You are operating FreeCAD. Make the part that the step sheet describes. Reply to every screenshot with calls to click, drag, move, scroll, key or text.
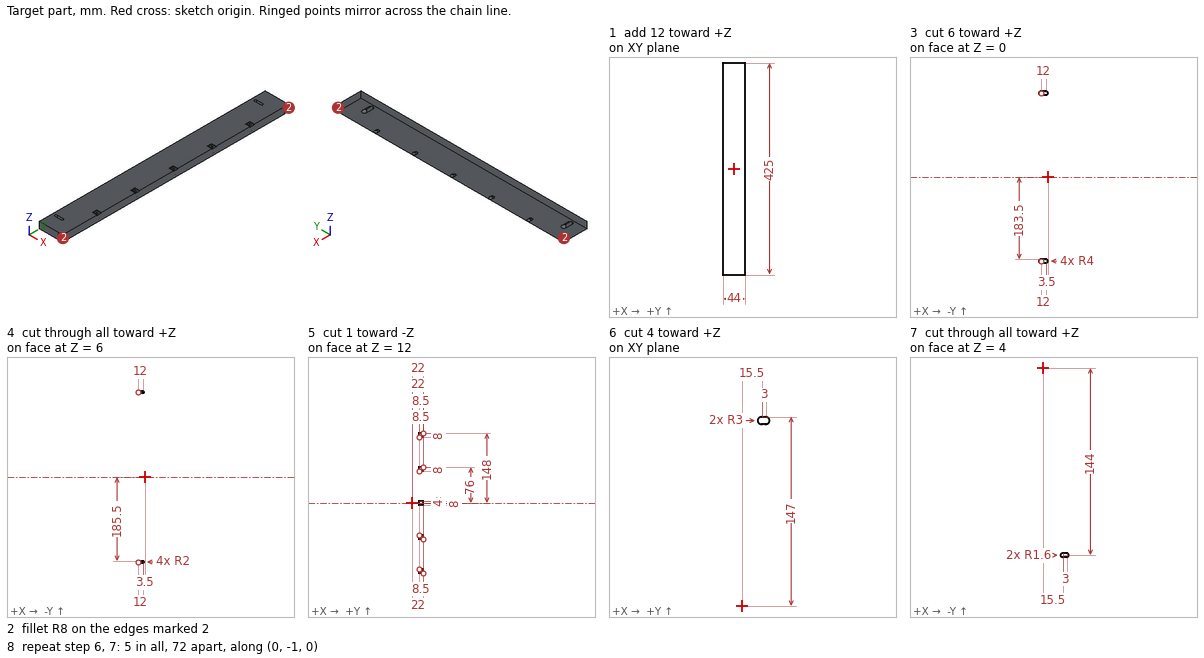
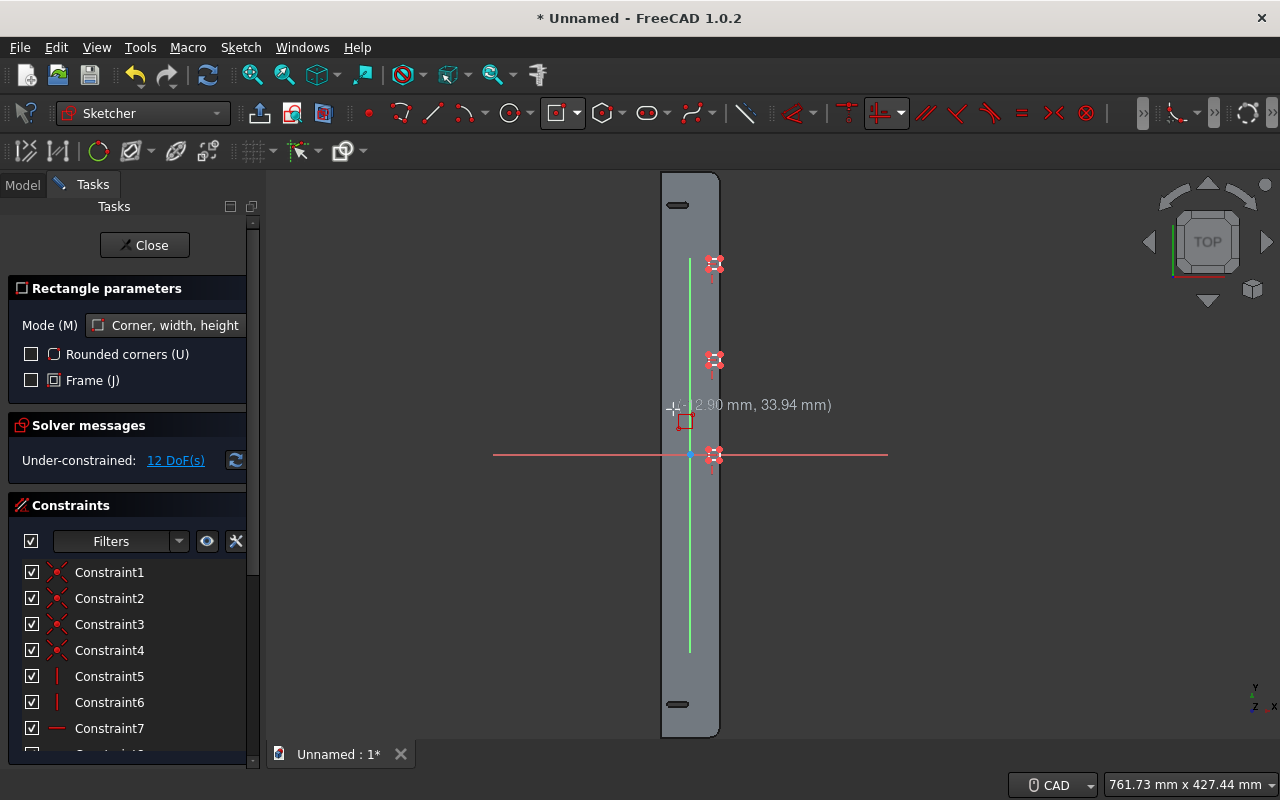
scroll(708, 545, up, 2)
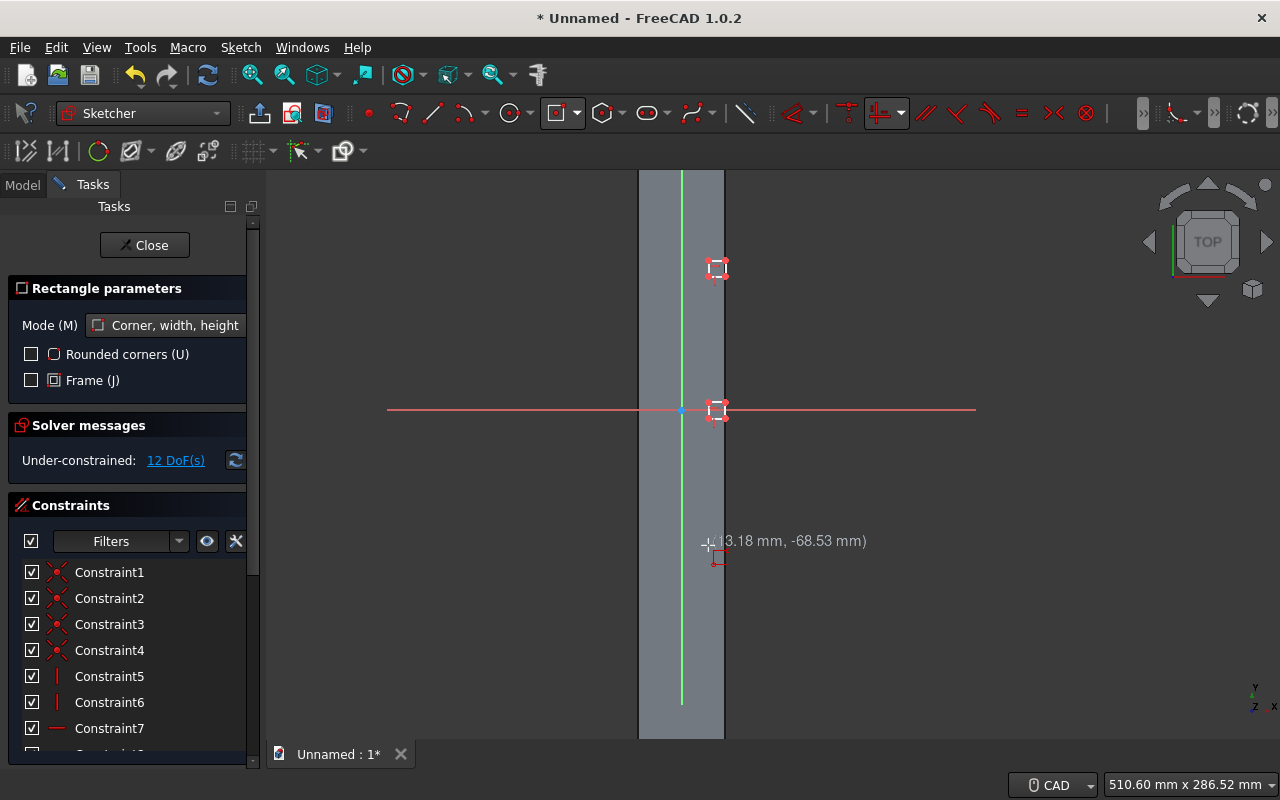
click(708, 545)
click(725, 561)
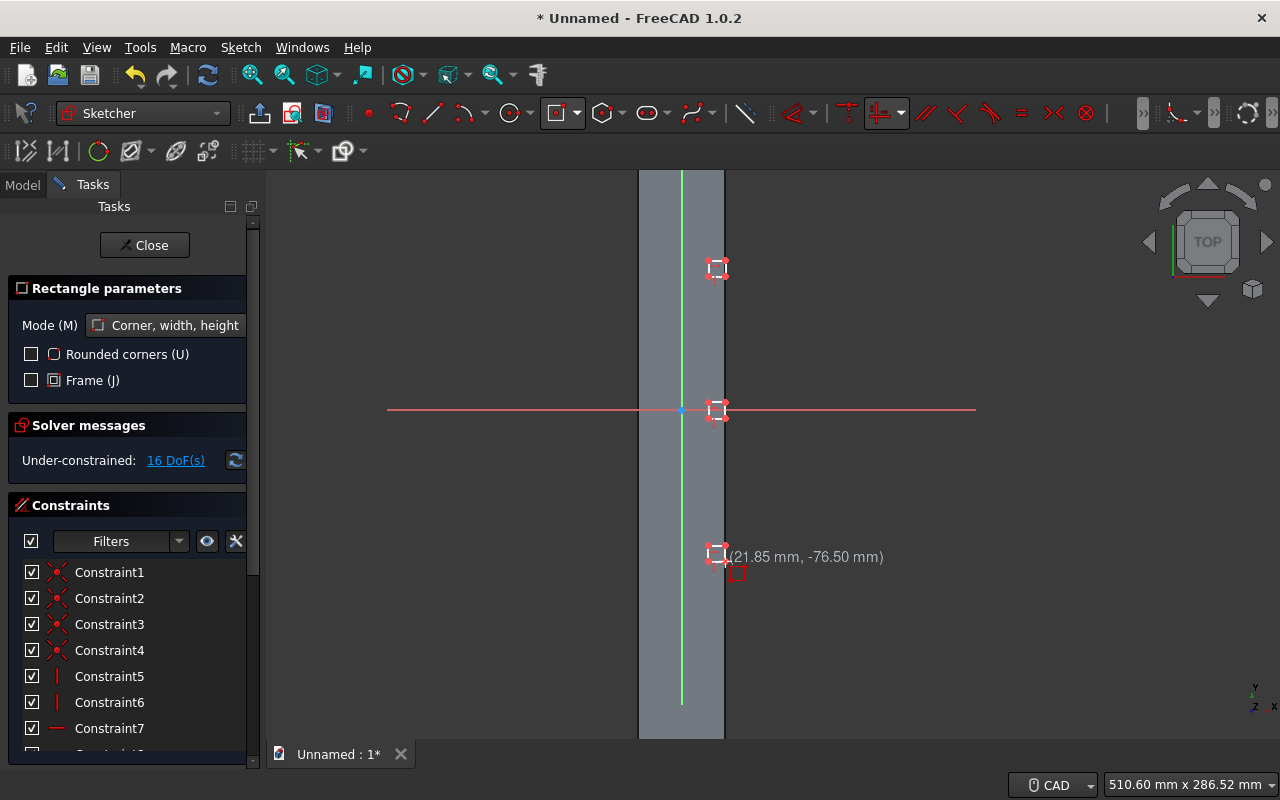
click(708, 688)
click(725, 704)
key(Escape)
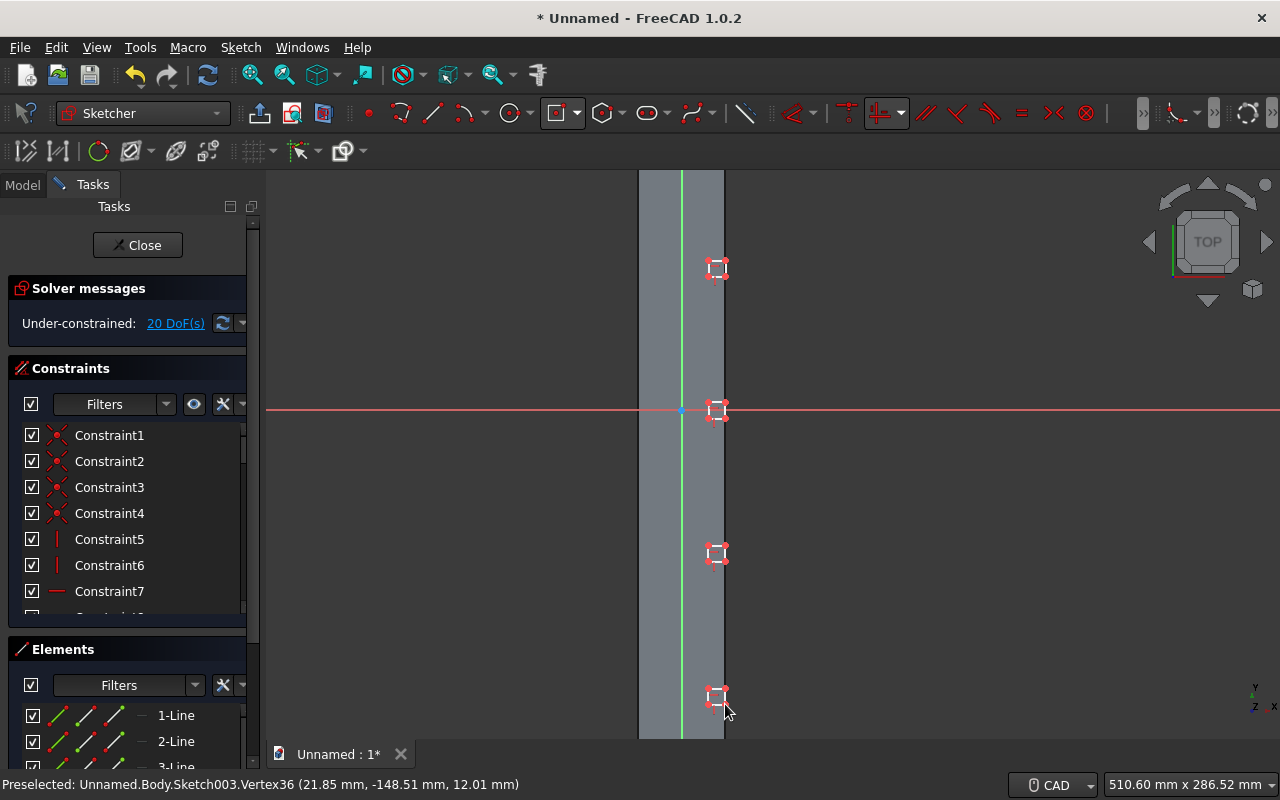
click(709, 277)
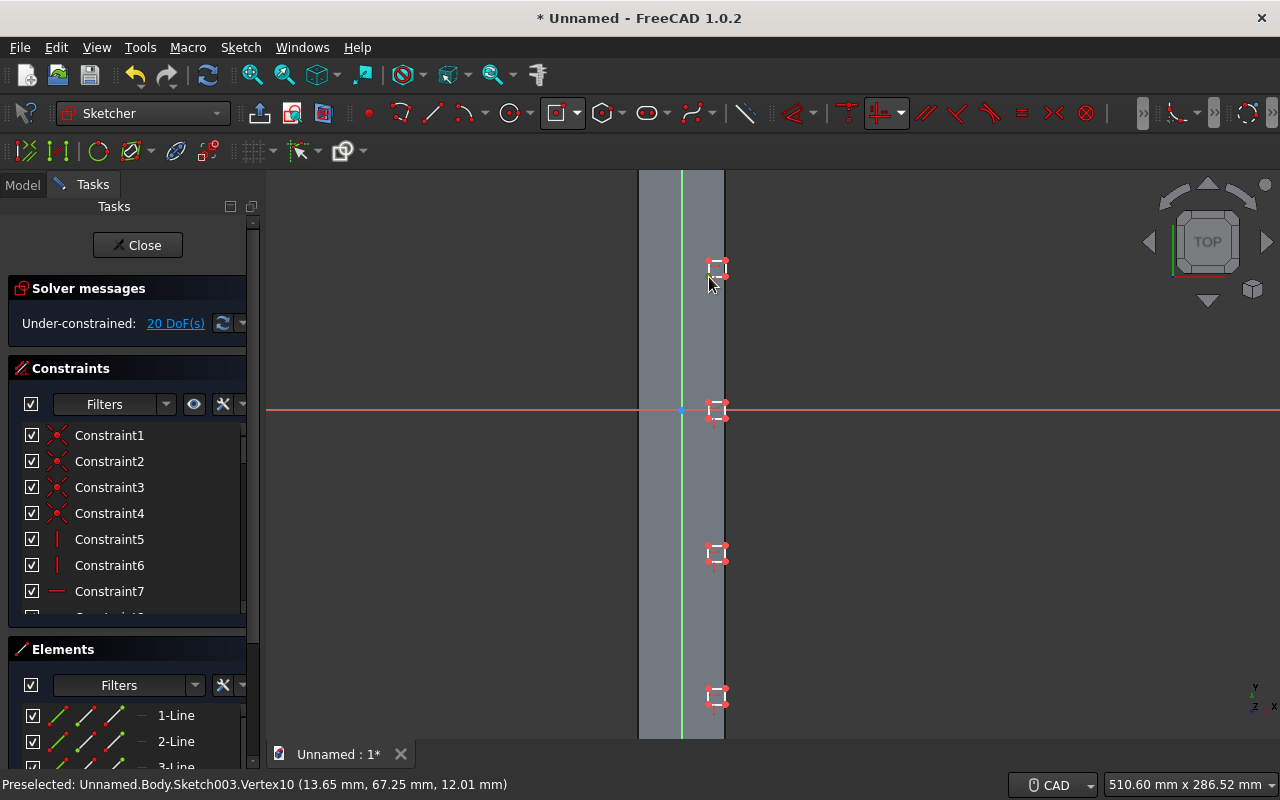
click(708, 546)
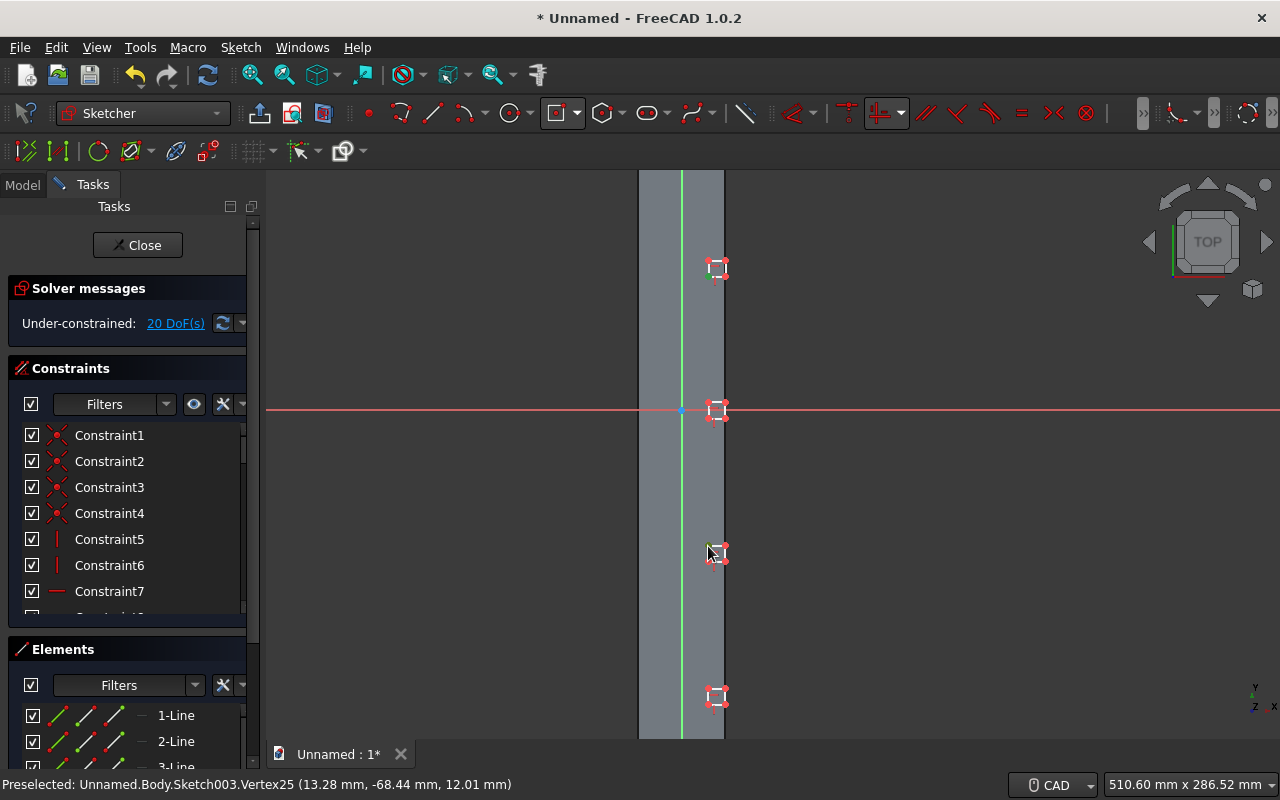
click(353, 410)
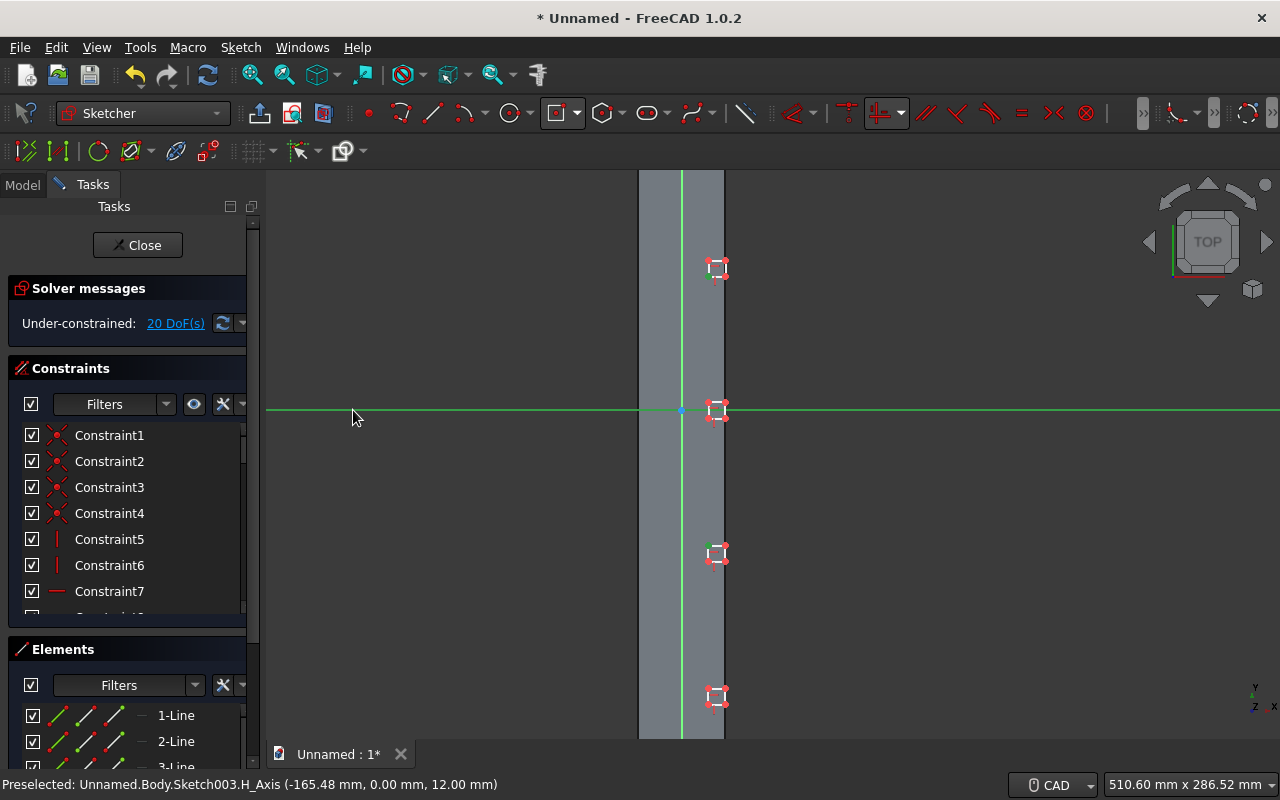
key(s)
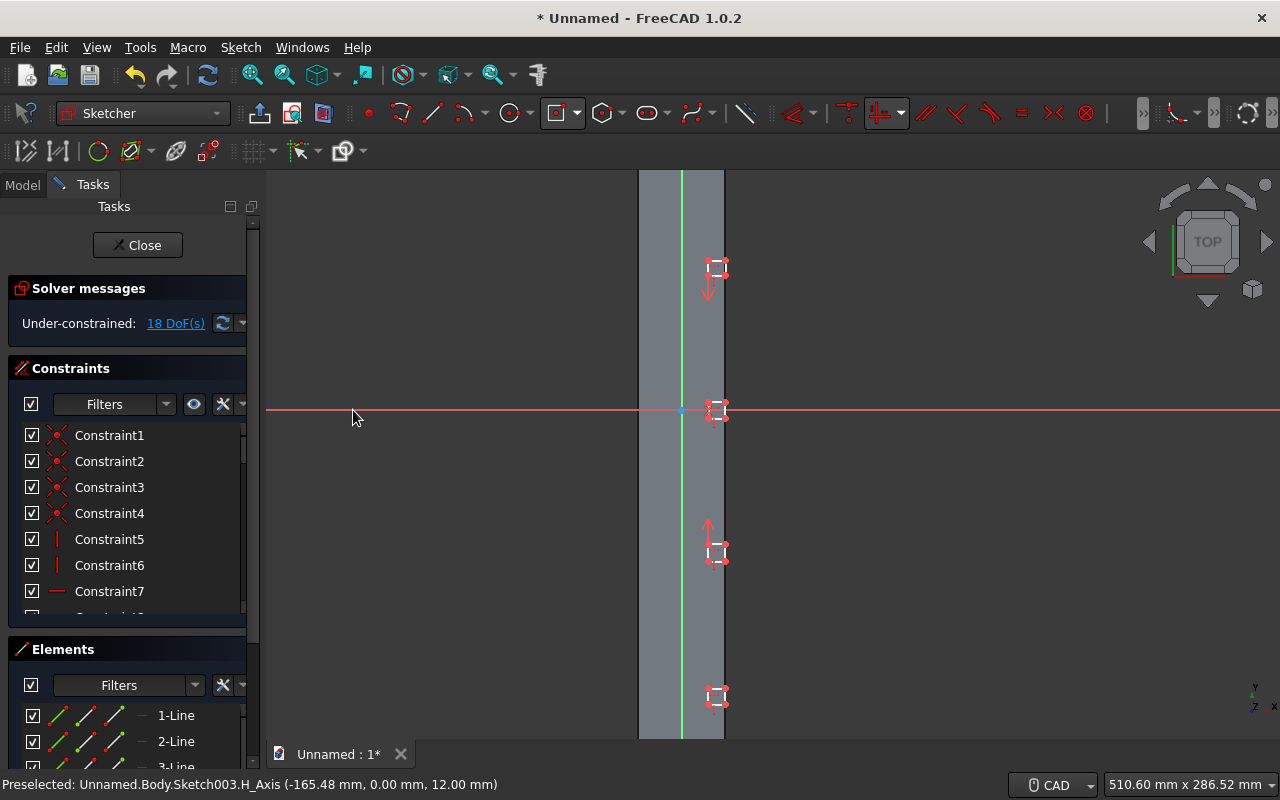
click(726, 261)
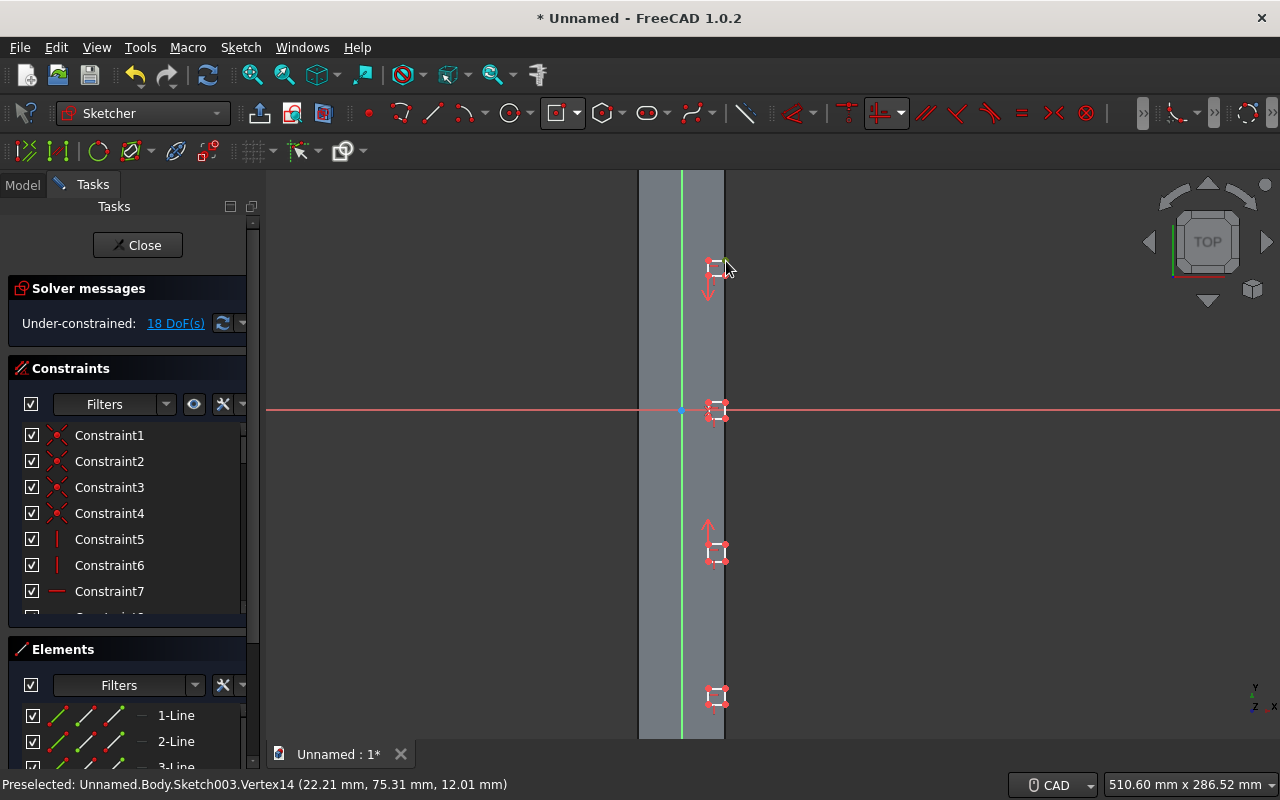
click(725, 562)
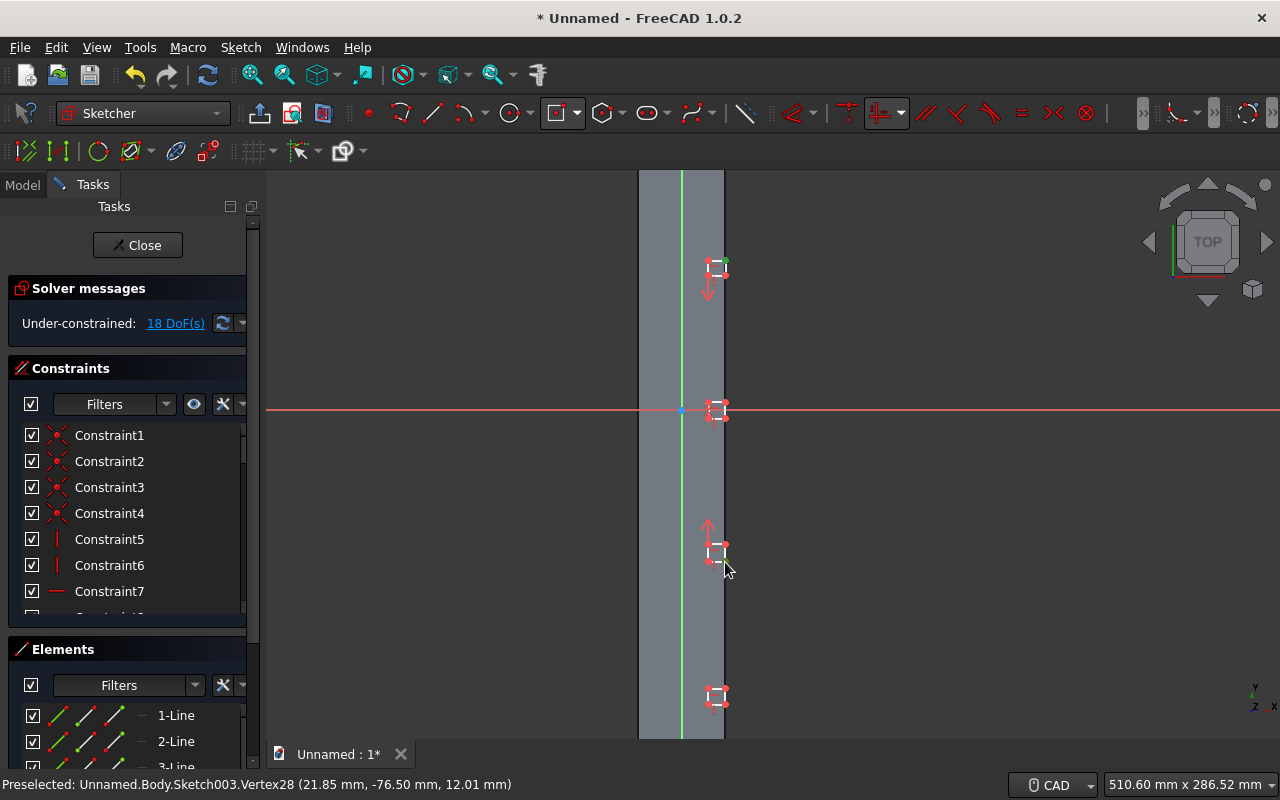
click(353, 410)